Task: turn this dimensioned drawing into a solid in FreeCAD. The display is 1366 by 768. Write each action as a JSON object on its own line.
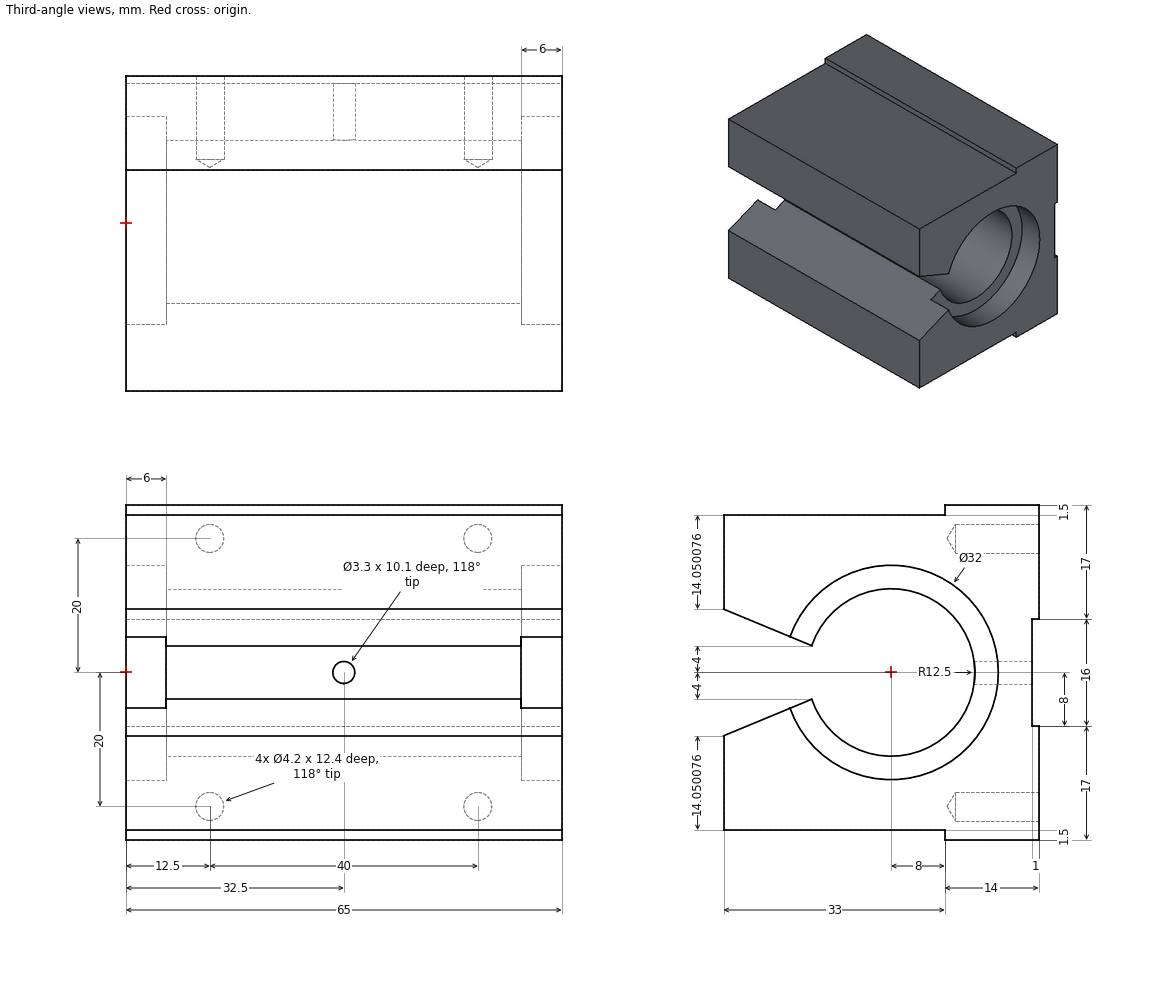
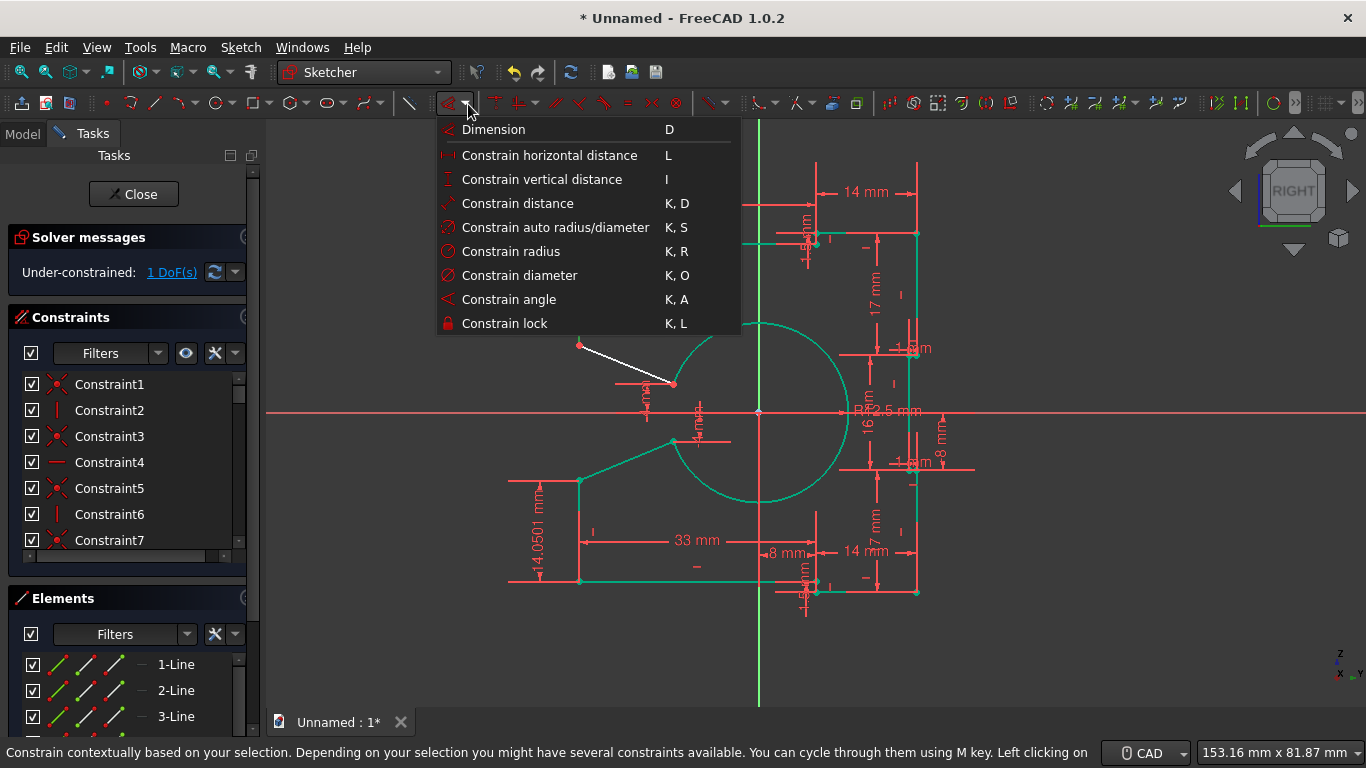
{"action": "left_click", "coordinate": [589, 179]}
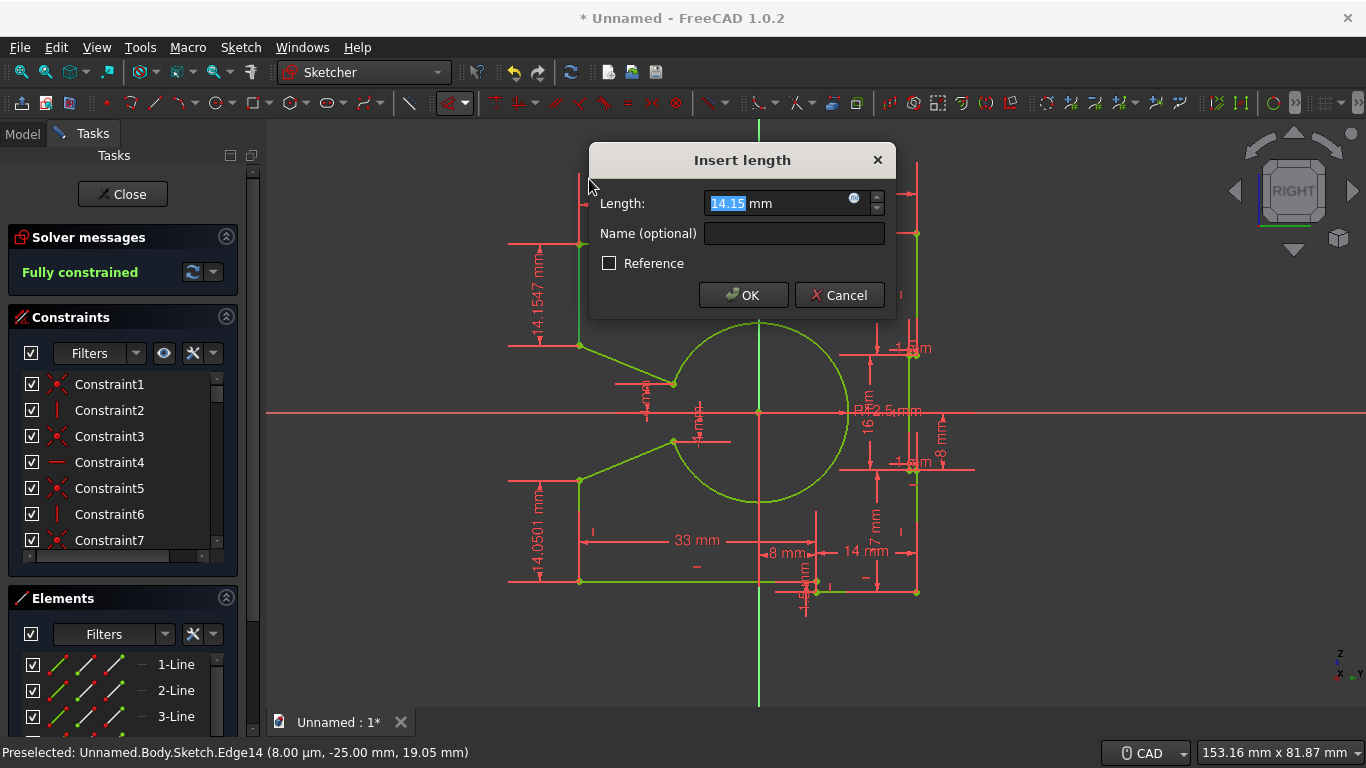
{"action": "type", "text": "14.050076"}
{"action": "key", "text": "Return"}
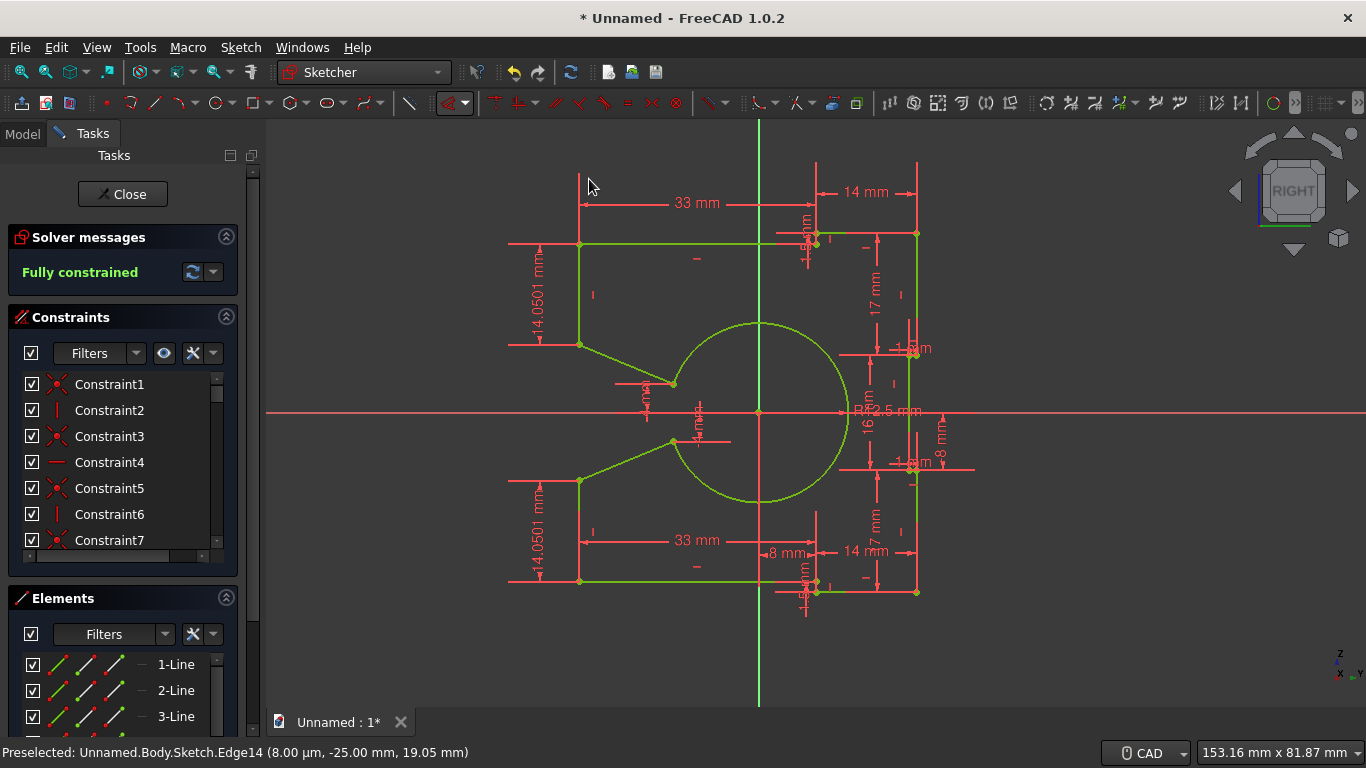
{"action": "left_click", "coordinate": [123, 194]}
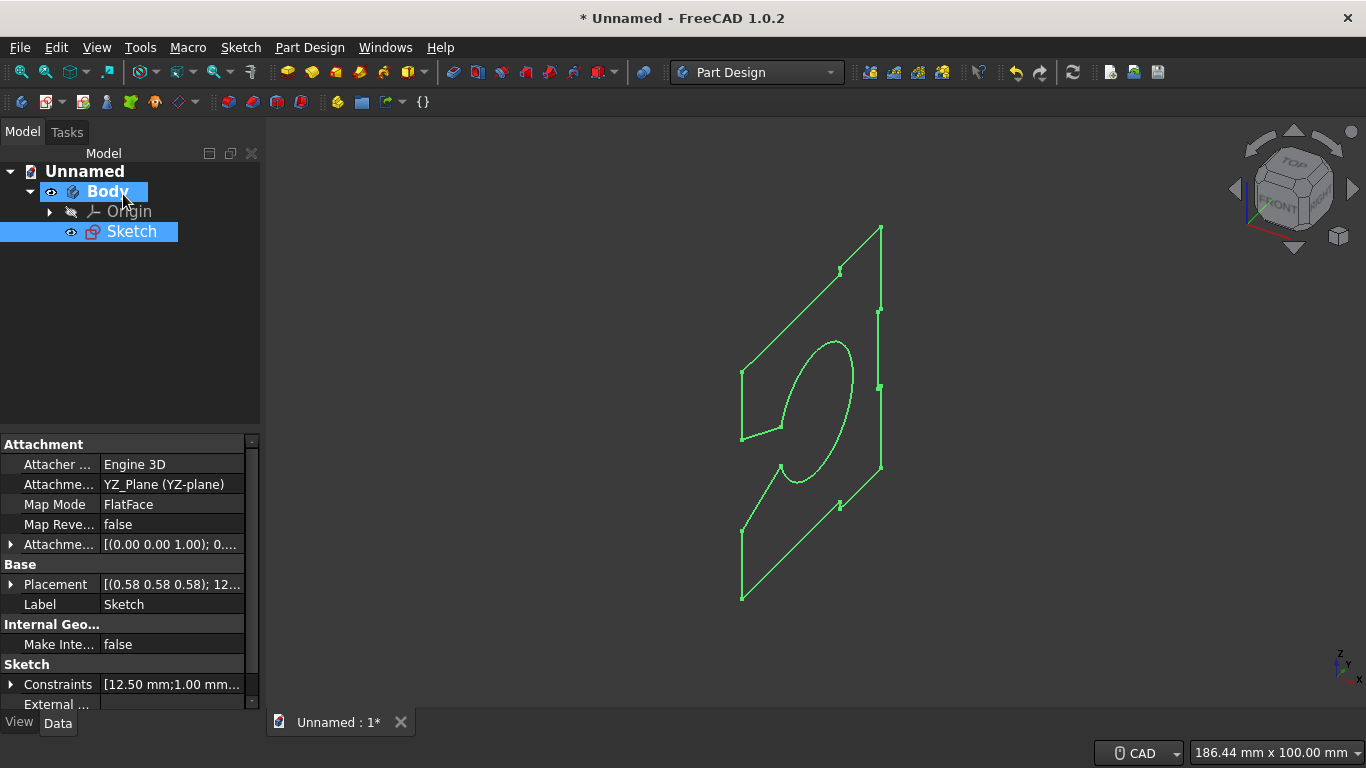
{"action": "left_click", "coordinate": [288, 72]}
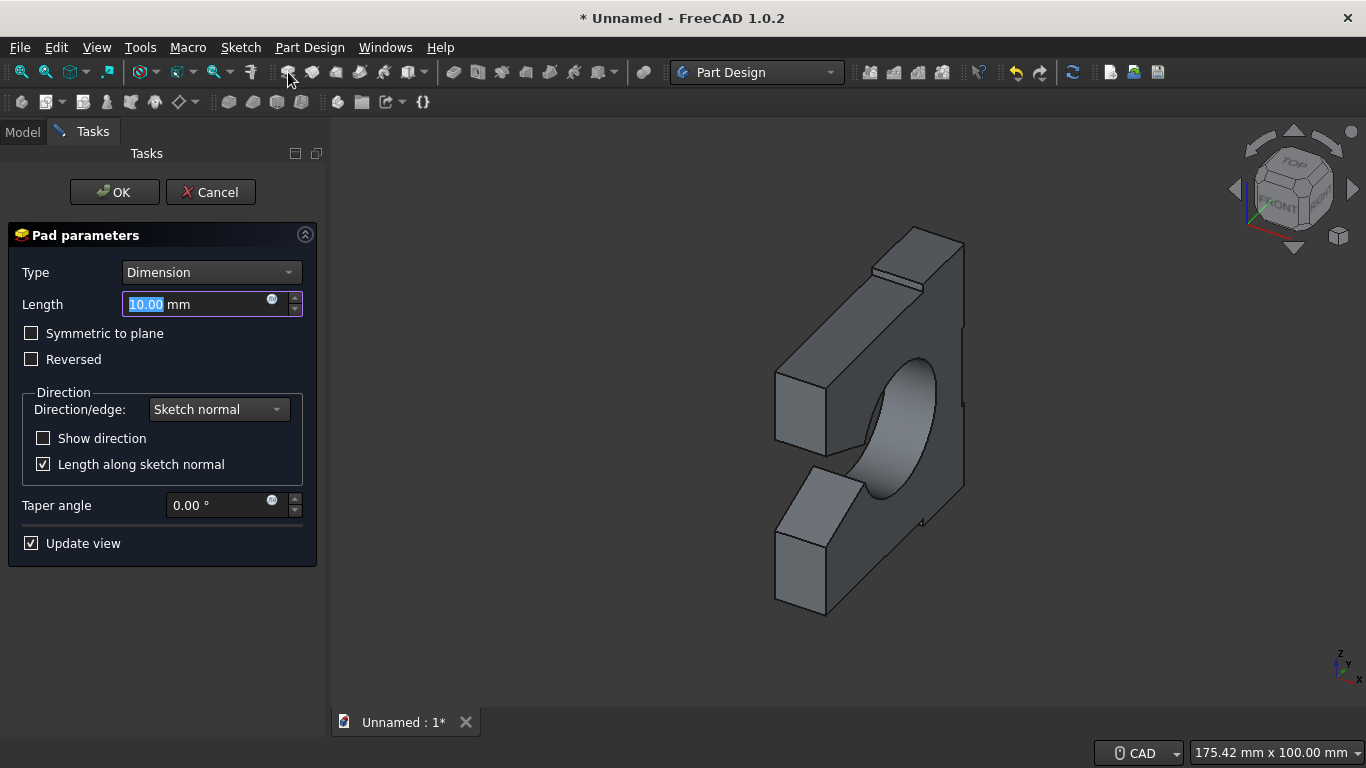
{"action": "type", "text": "65"}
{"action": "key", "text": "Tab"}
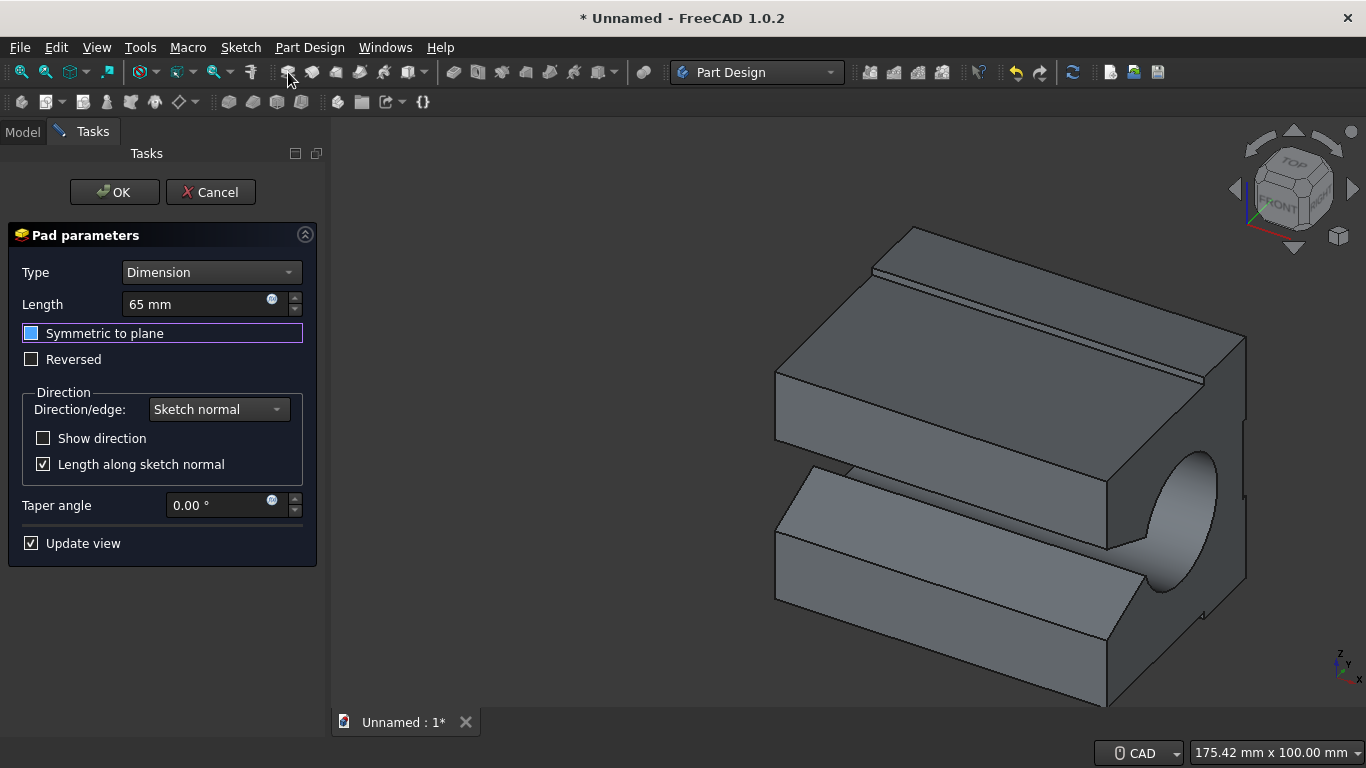
{"action": "left_click", "coordinate": [115, 192]}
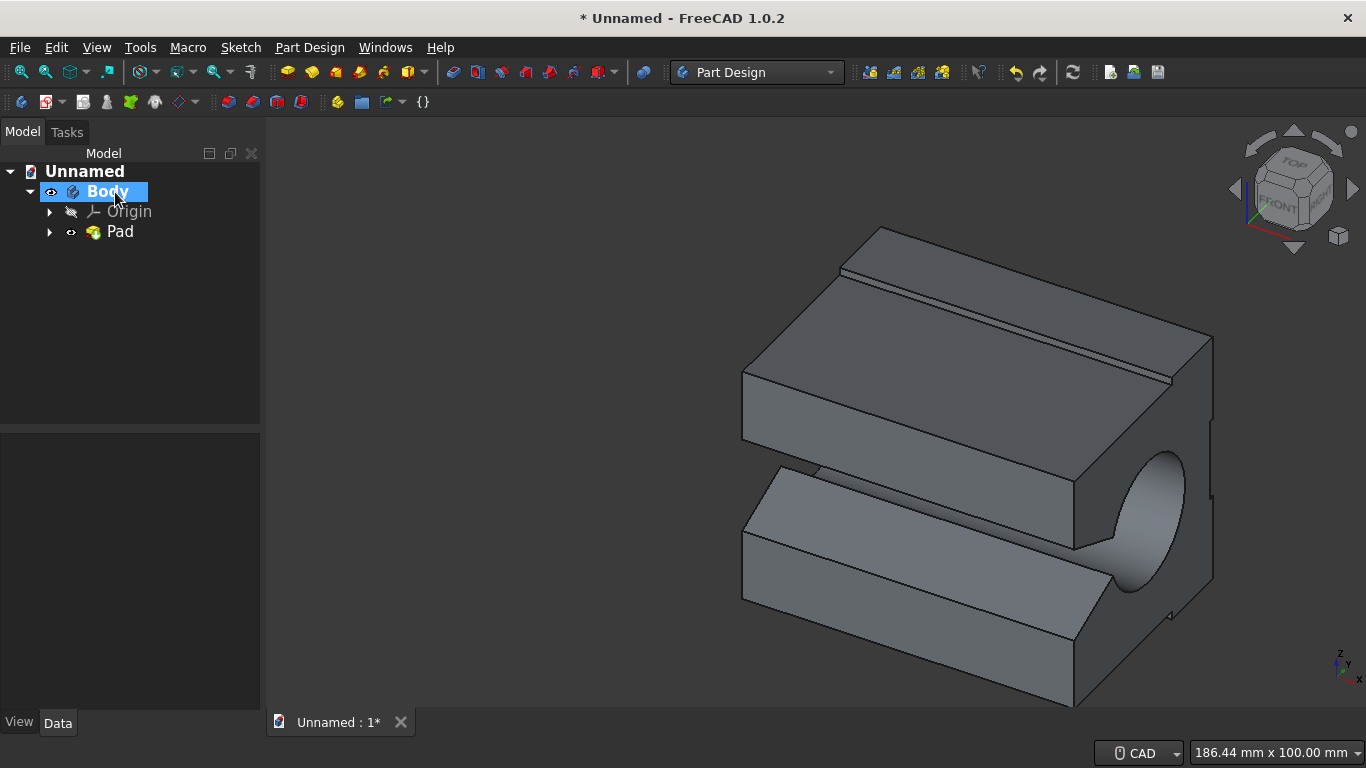
{"action": "left_click", "coordinate": [22, 72]}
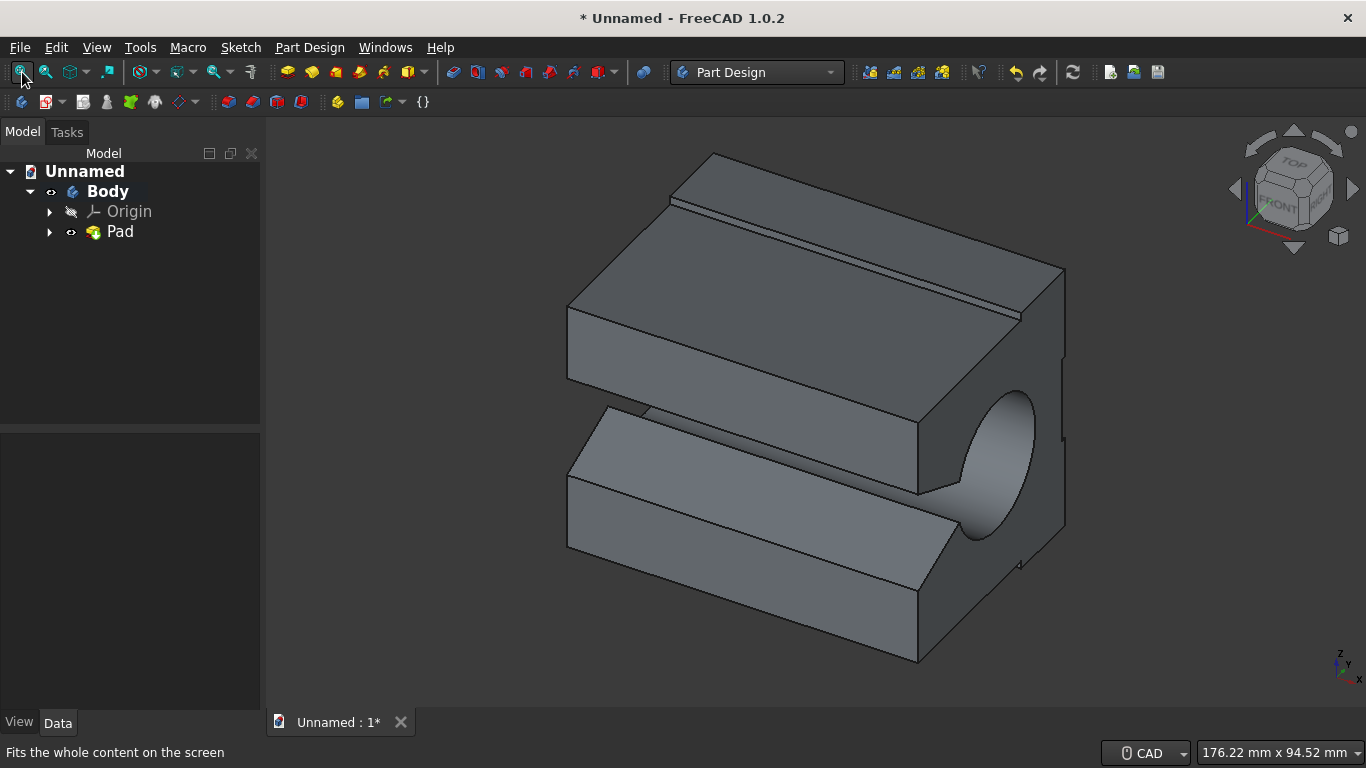
{"action": "left_click", "coordinate": [950, 438]}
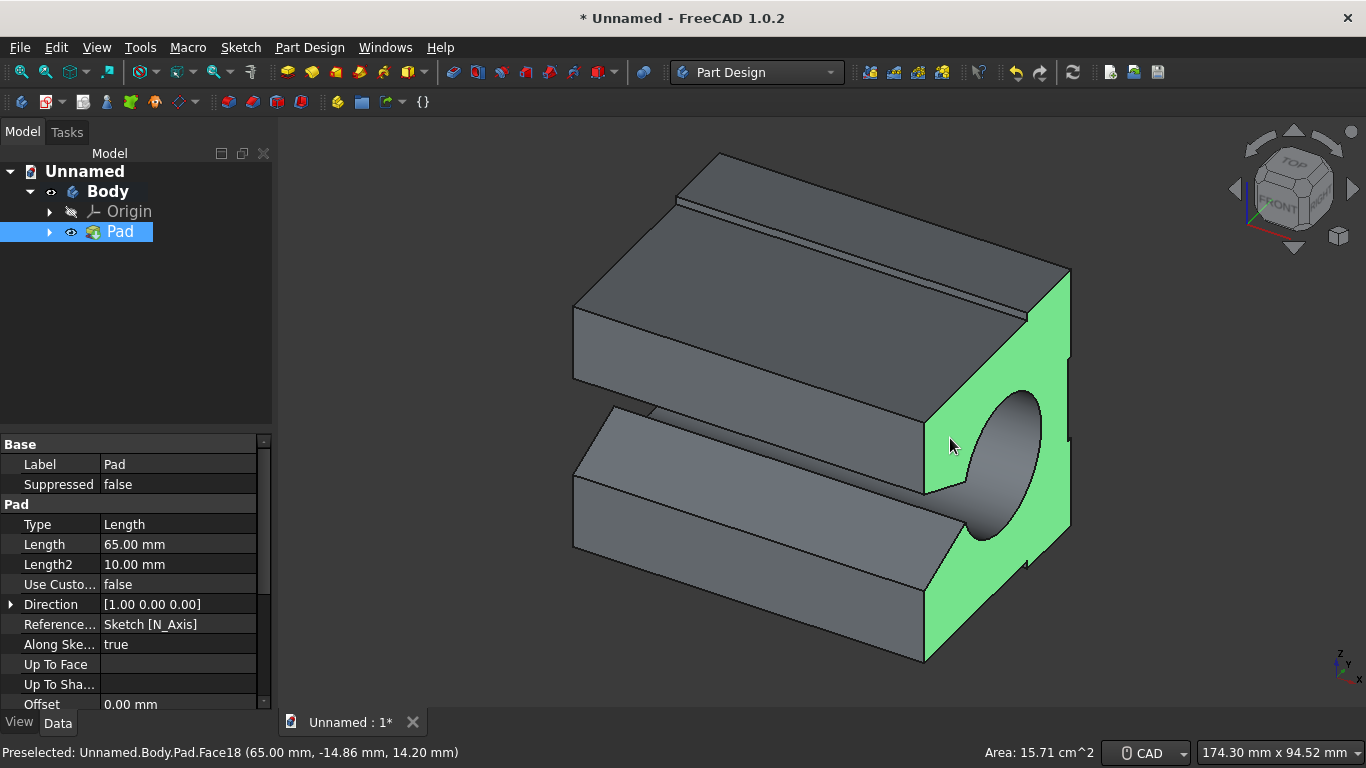
{"action": "left_click", "coordinate": [46, 102]}